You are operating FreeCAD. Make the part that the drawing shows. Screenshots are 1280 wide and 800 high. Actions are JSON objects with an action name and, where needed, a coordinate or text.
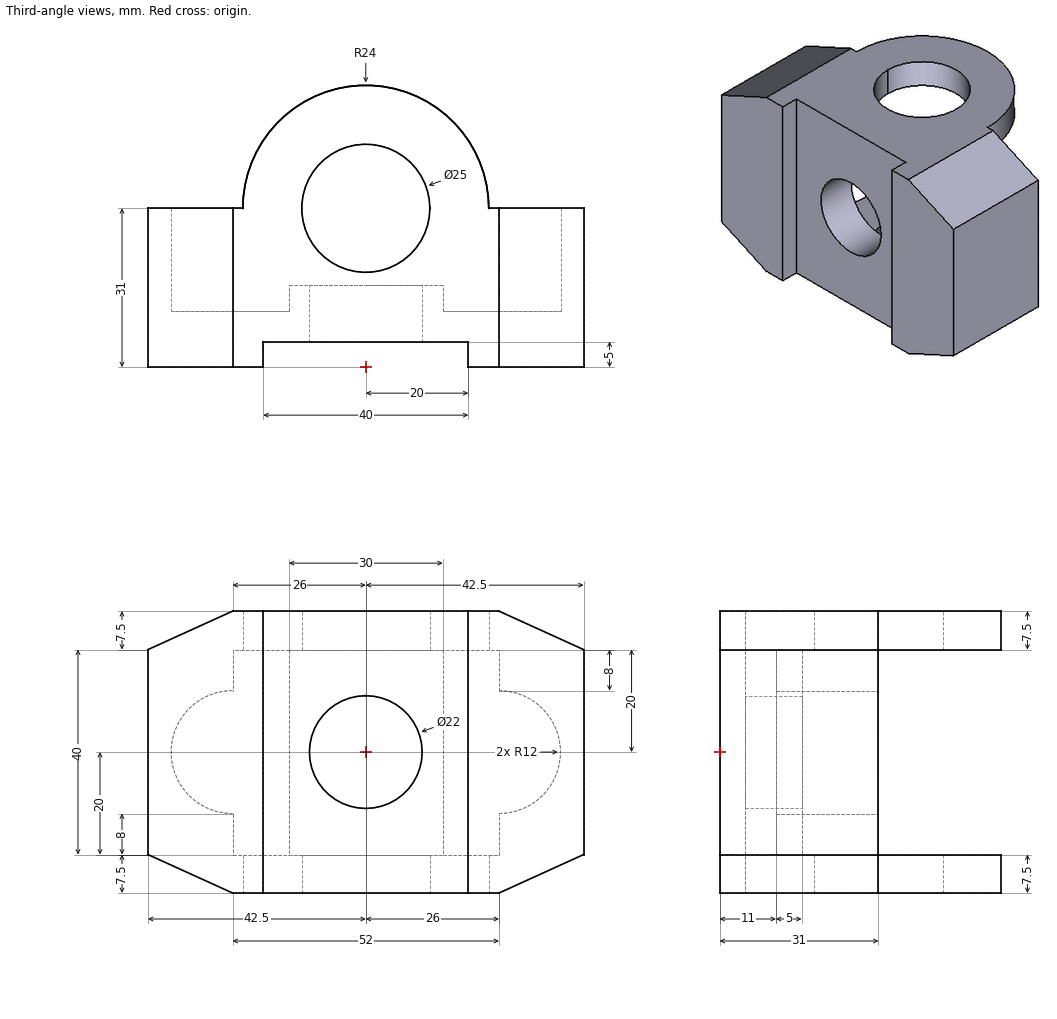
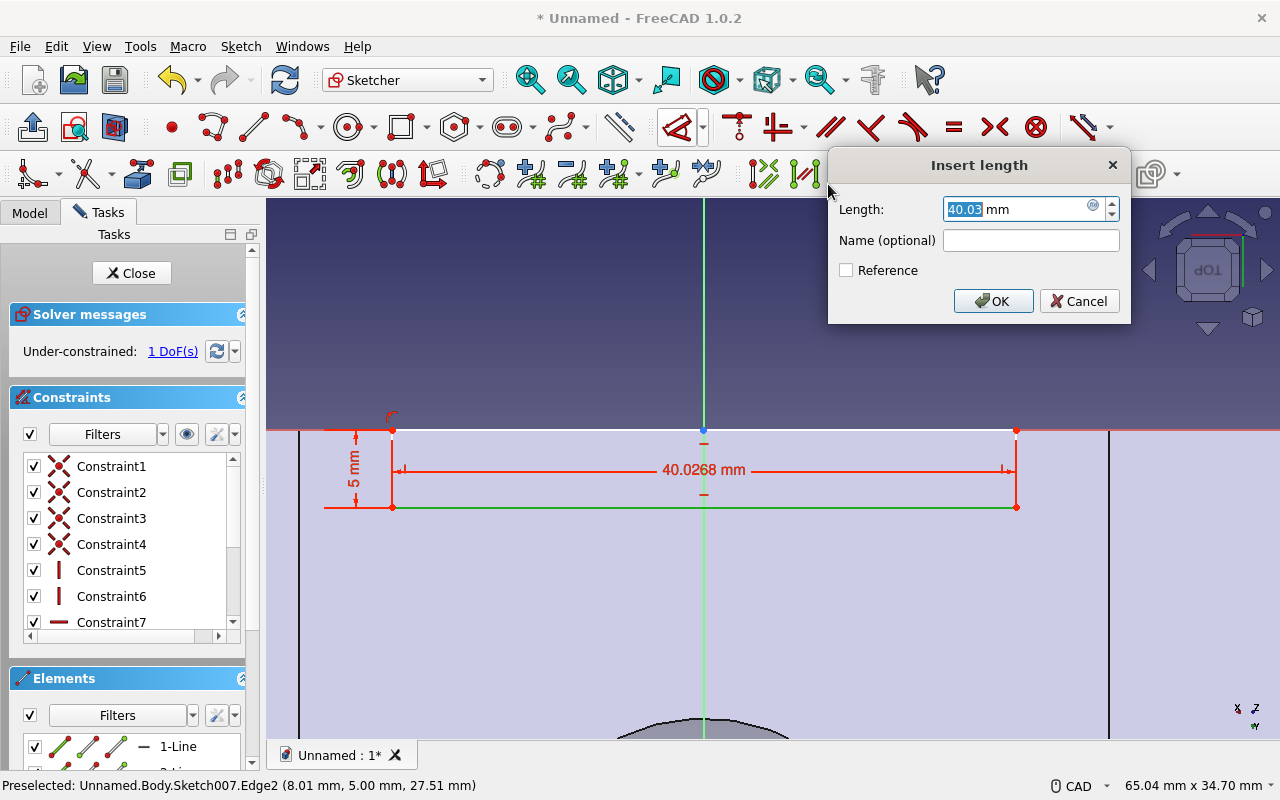
{"action": "type", "text": "40"}
{"action": "key", "text": "Return"}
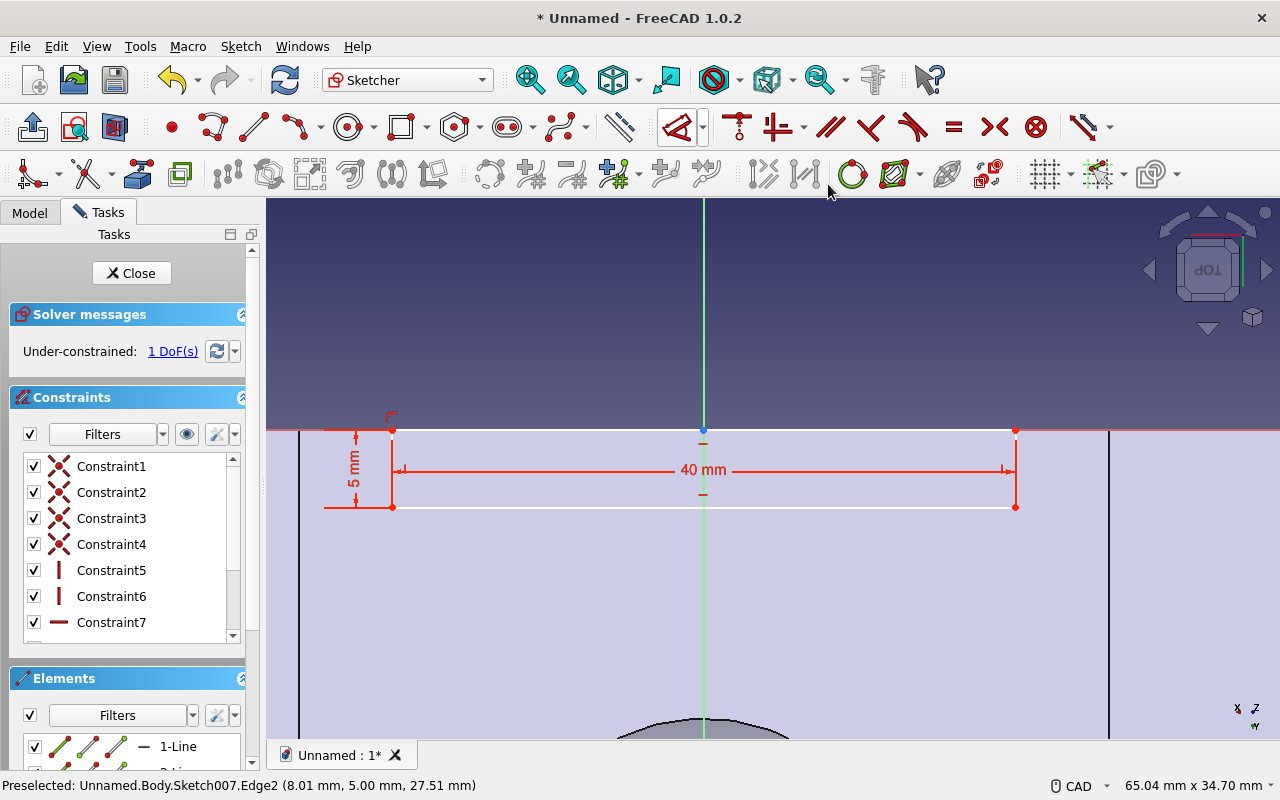
{"action": "left_click", "coordinate": [392, 430]}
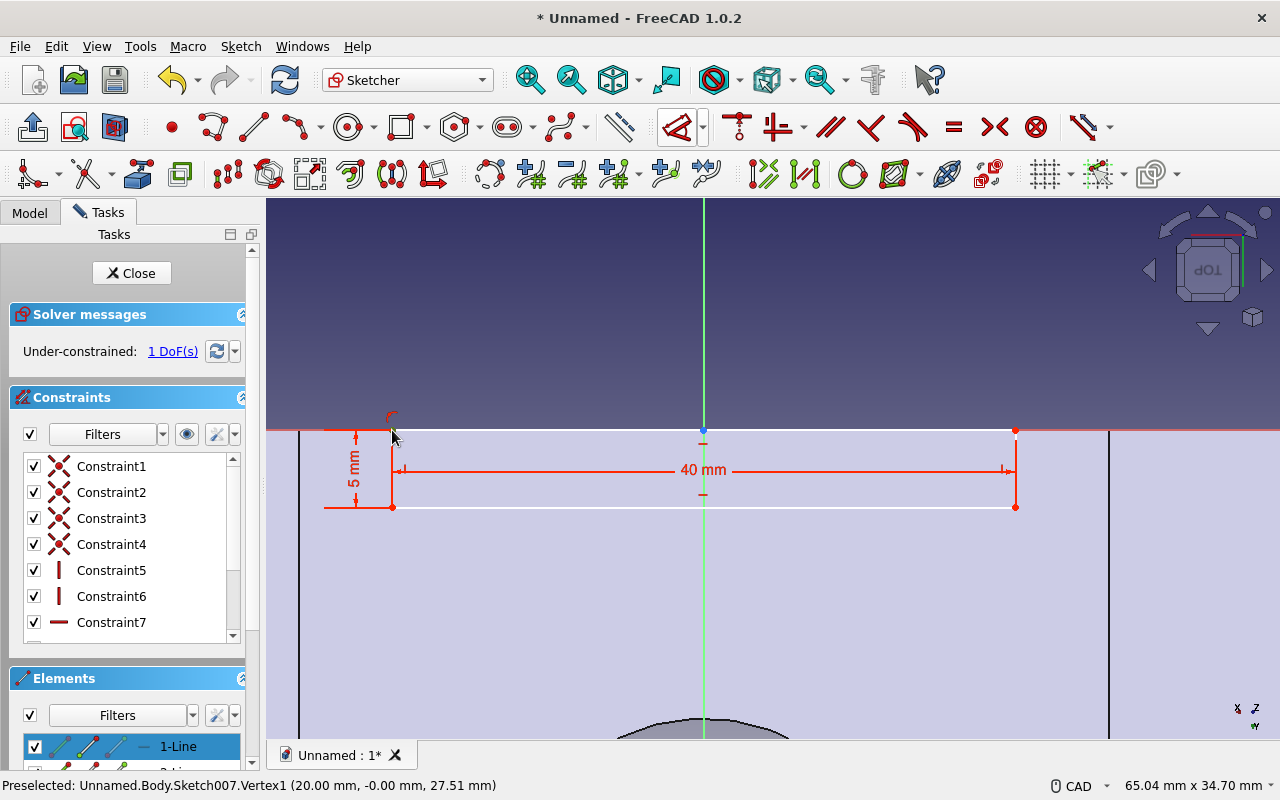
{"action": "key", "text": "l"}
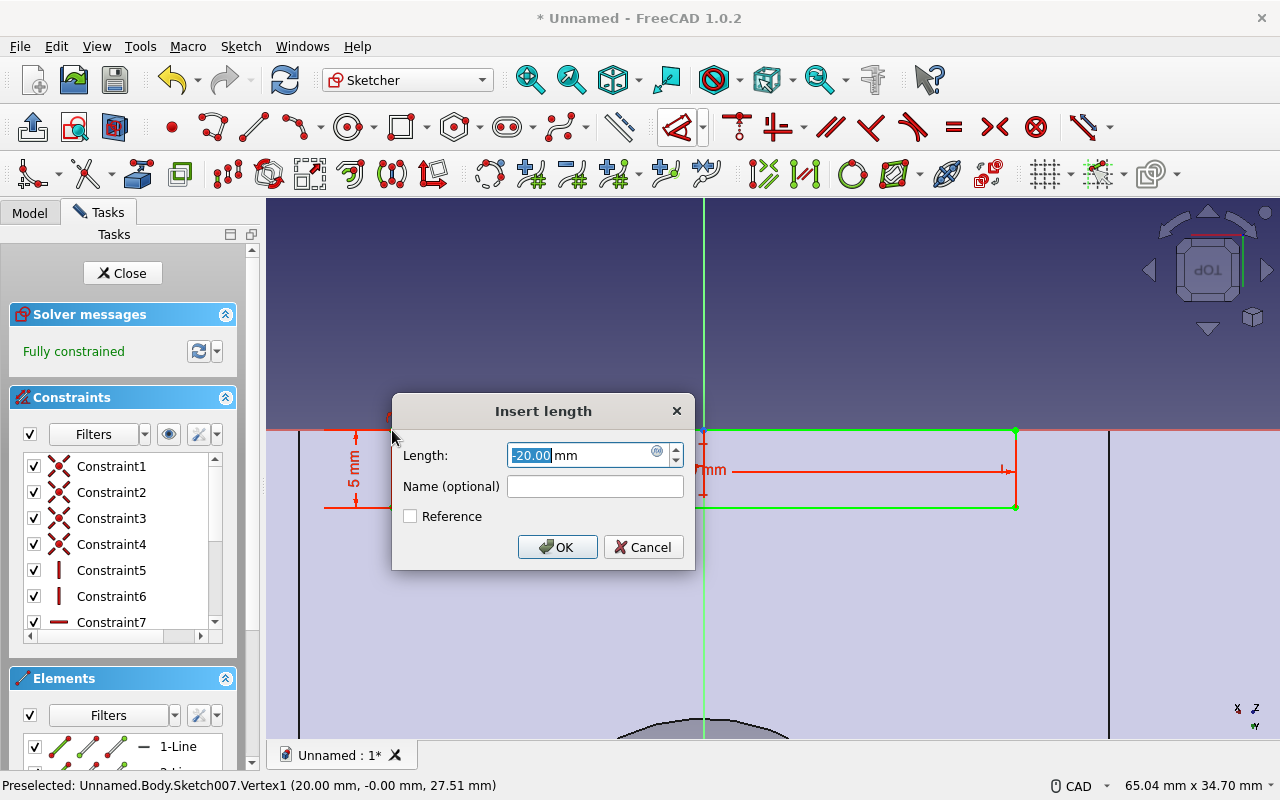
{"action": "type", "text": "-20"}
{"action": "key", "text": "Return"}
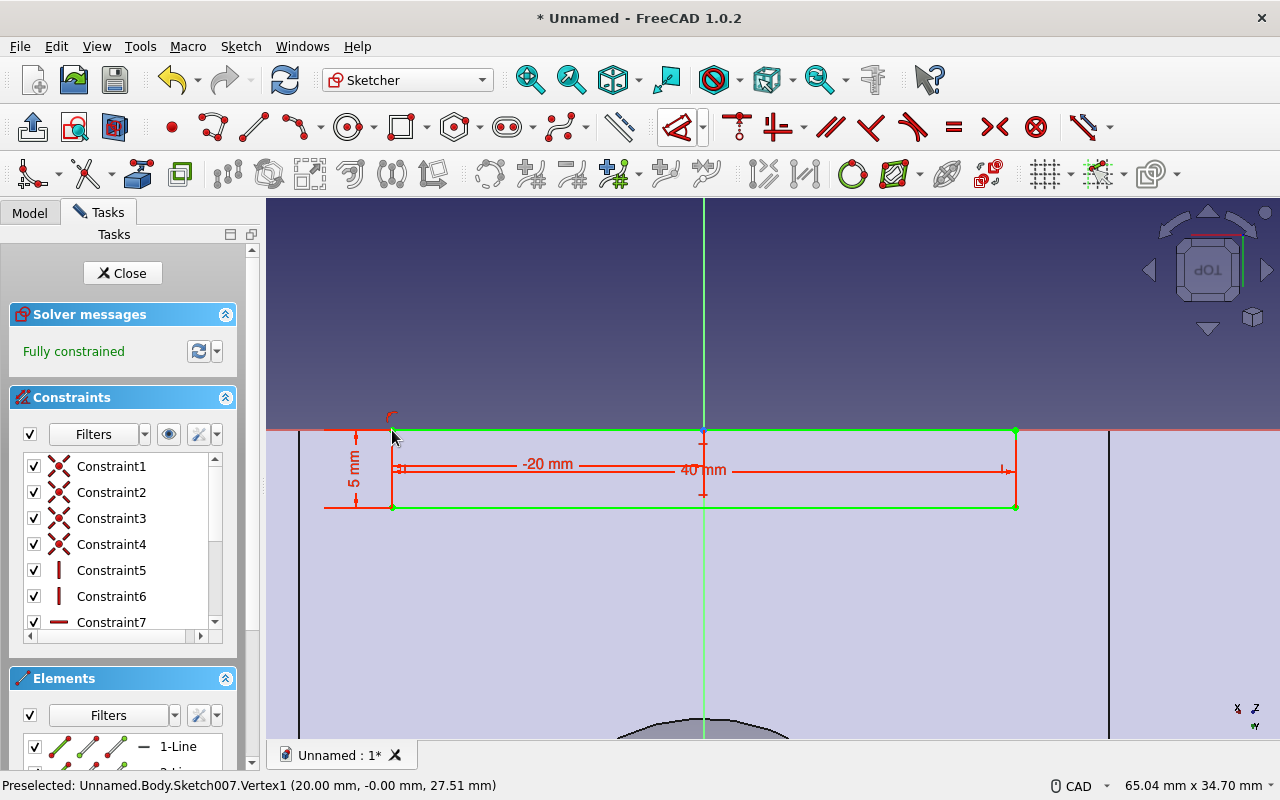
{"action": "left_click", "coordinate": [123, 273]}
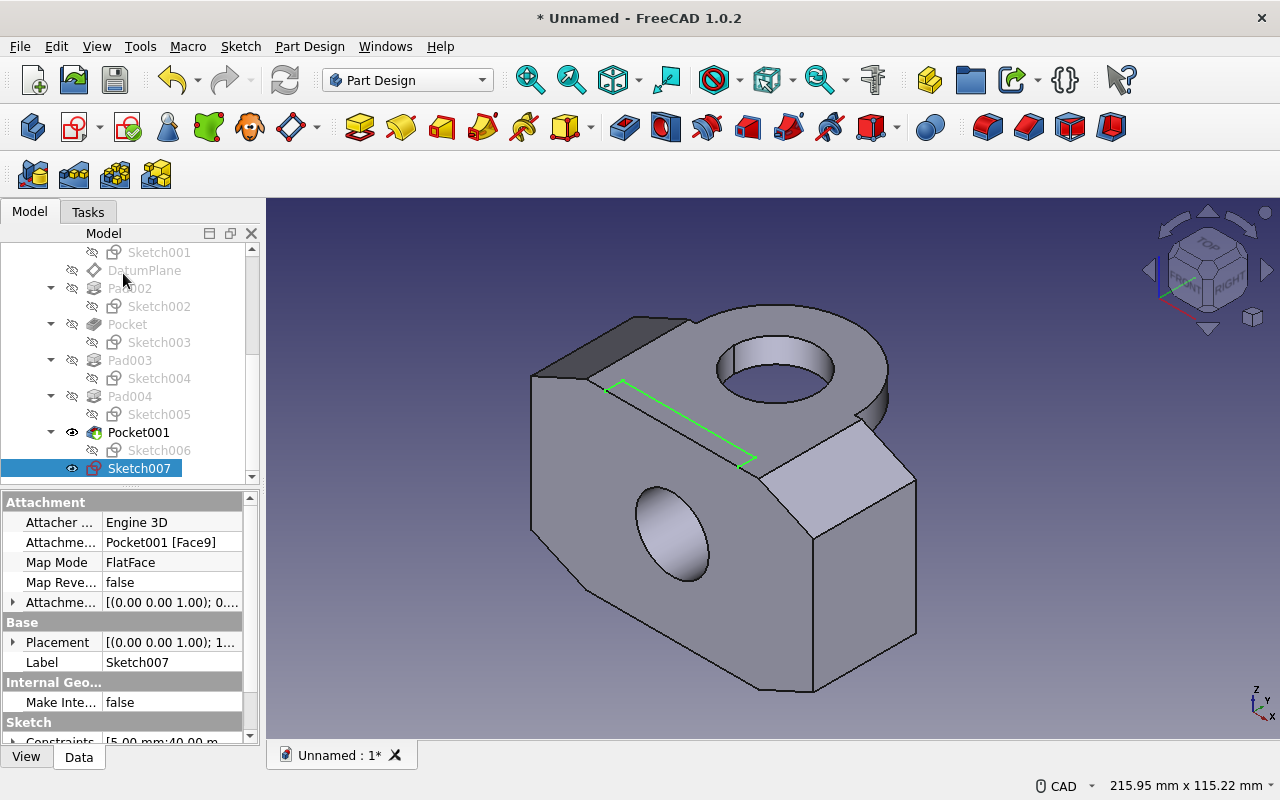
{"action": "left_click", "coordinate": [625, 128]}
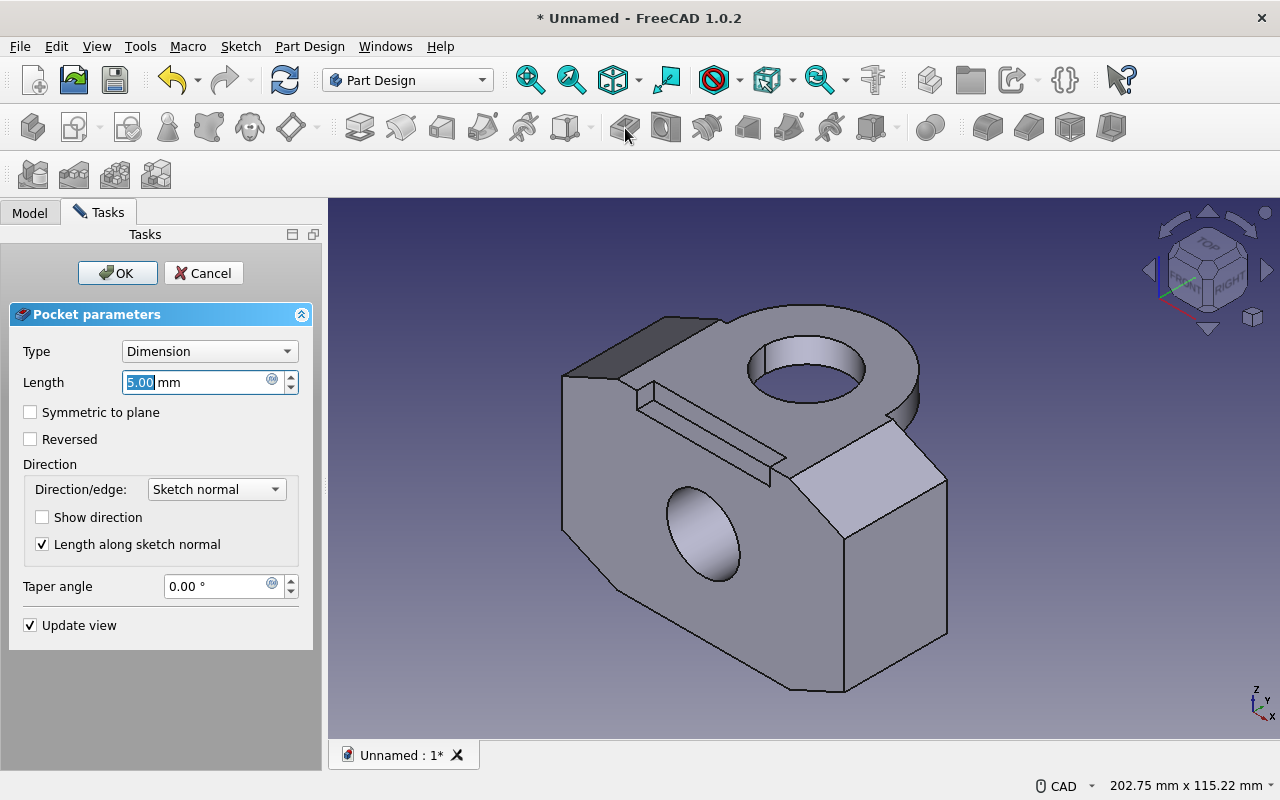
{"action": "left_click", "coordinate": [210, 352]}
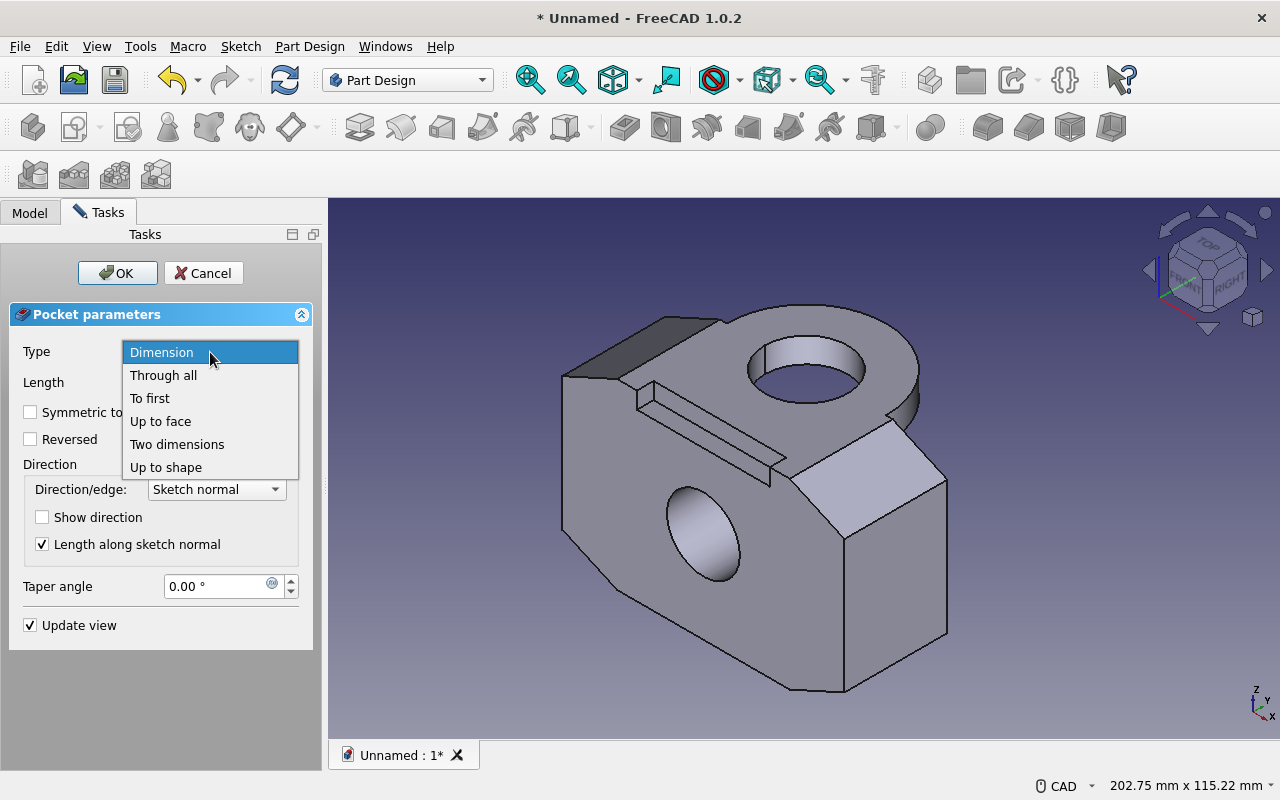
{"action": "left_click", "coordinate": [208, 398]}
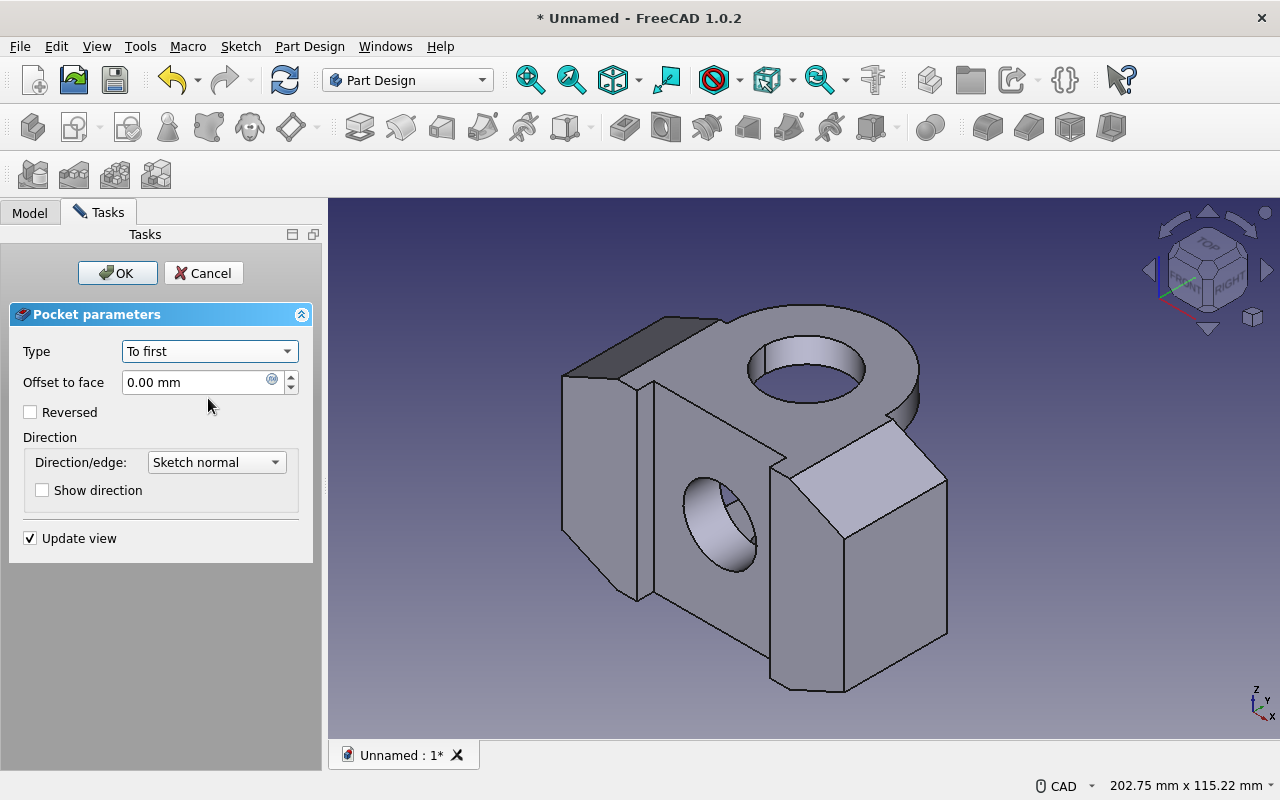
{"action": "left_click", "coordinate": [118, 273]}